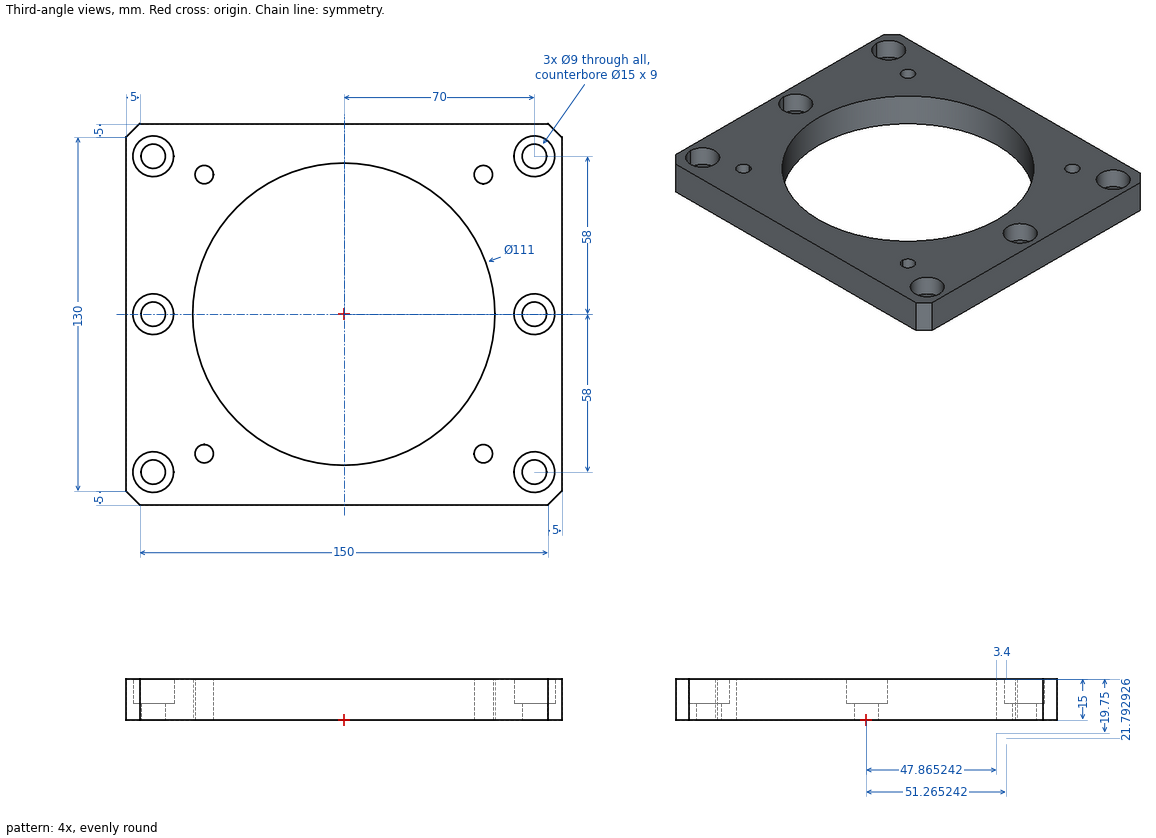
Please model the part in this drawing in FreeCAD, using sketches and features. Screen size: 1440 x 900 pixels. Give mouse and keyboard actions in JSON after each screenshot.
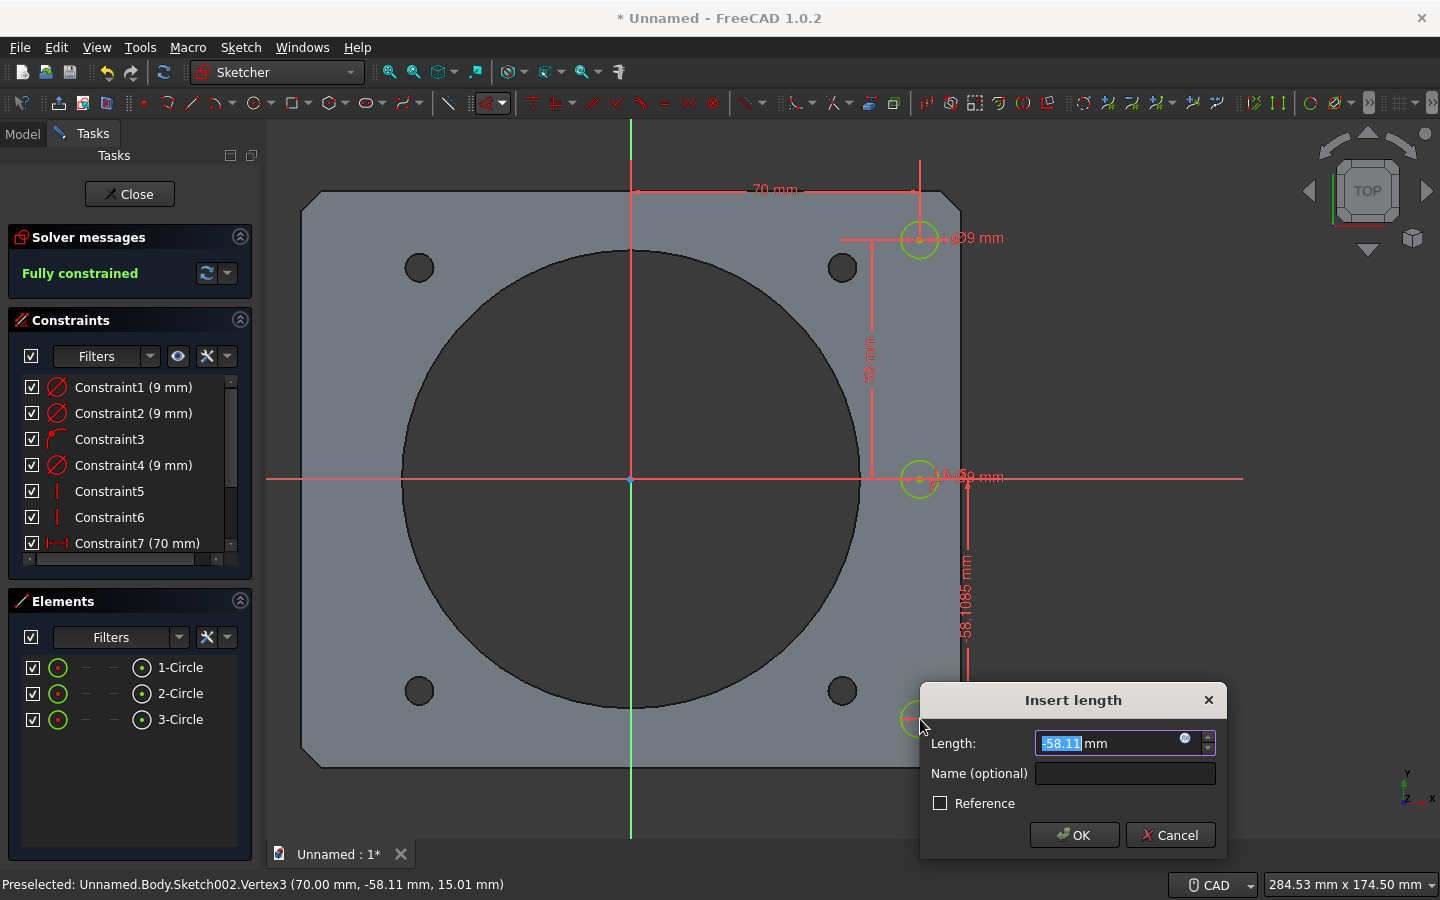
{"action": "type", "text": "-58"}
{"action": "key", "text": "Return"}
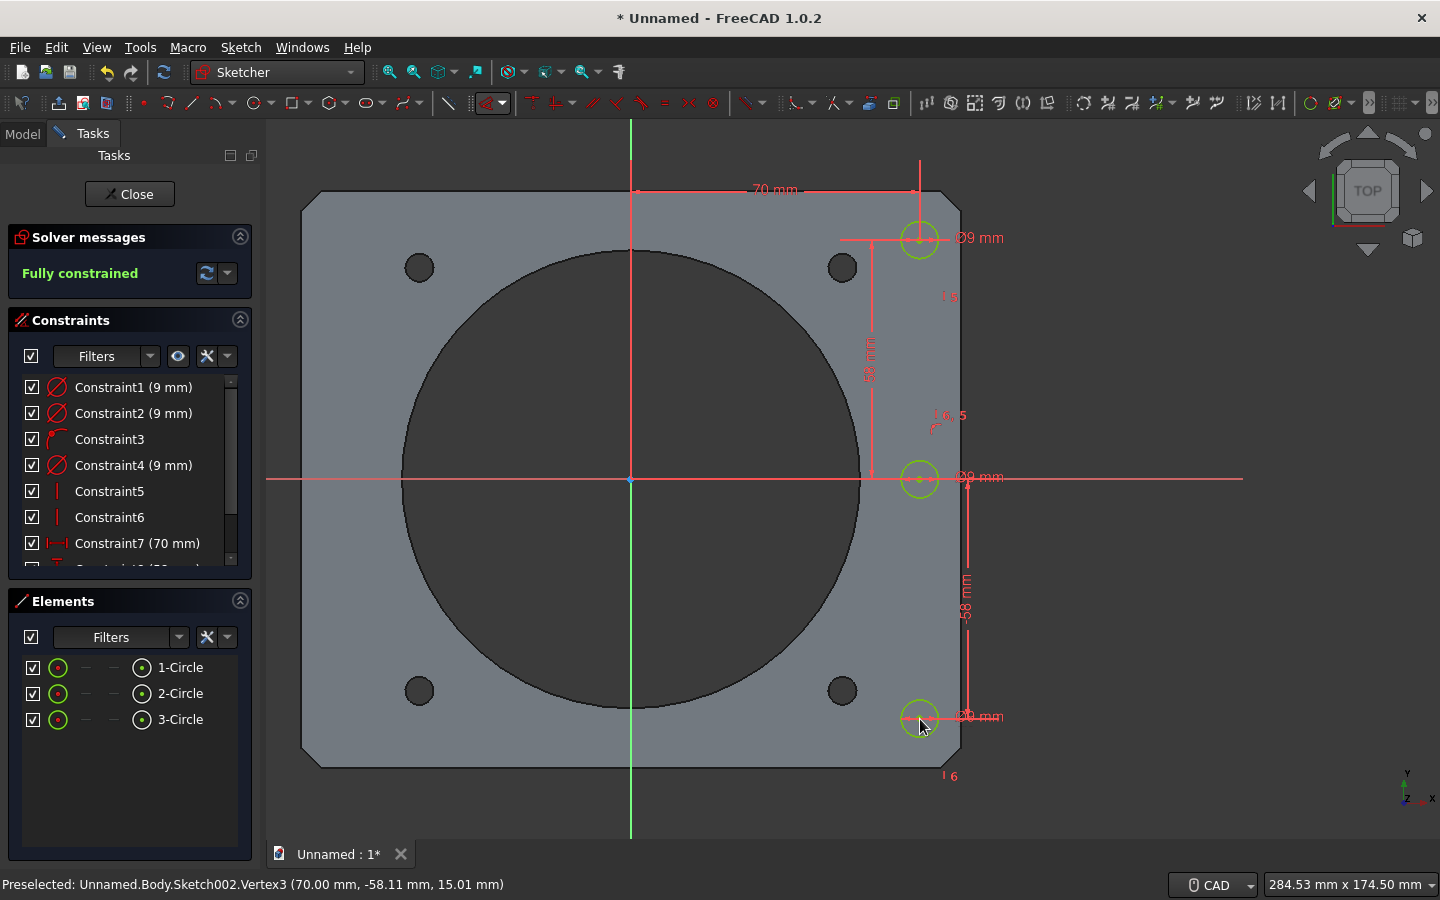
{"action": "left_click", "coordinate": [130, 194]}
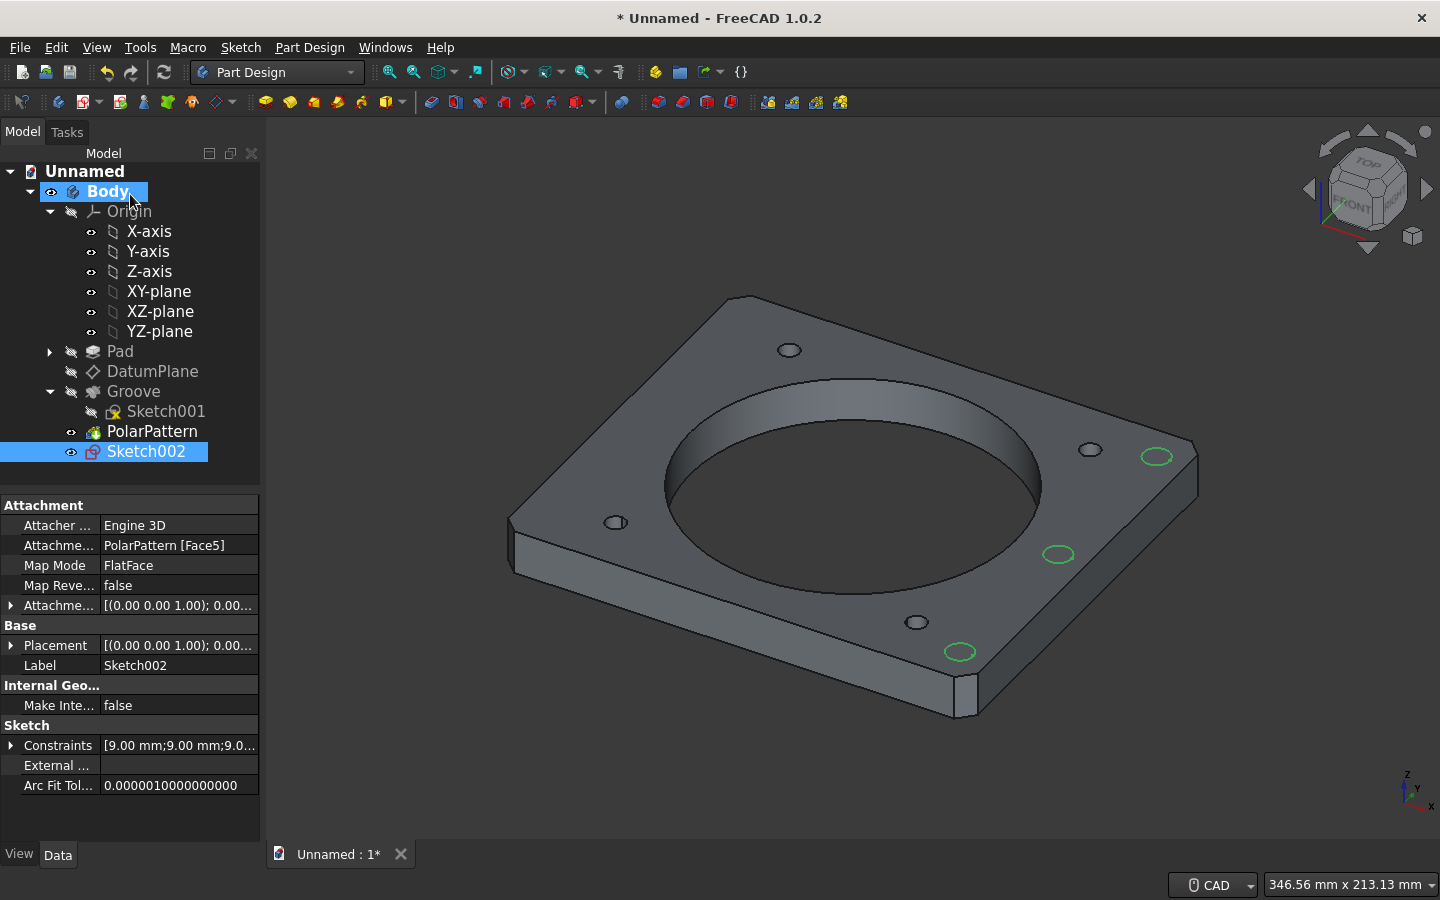
{"action": "left_click", "coordinate": [456, 102]}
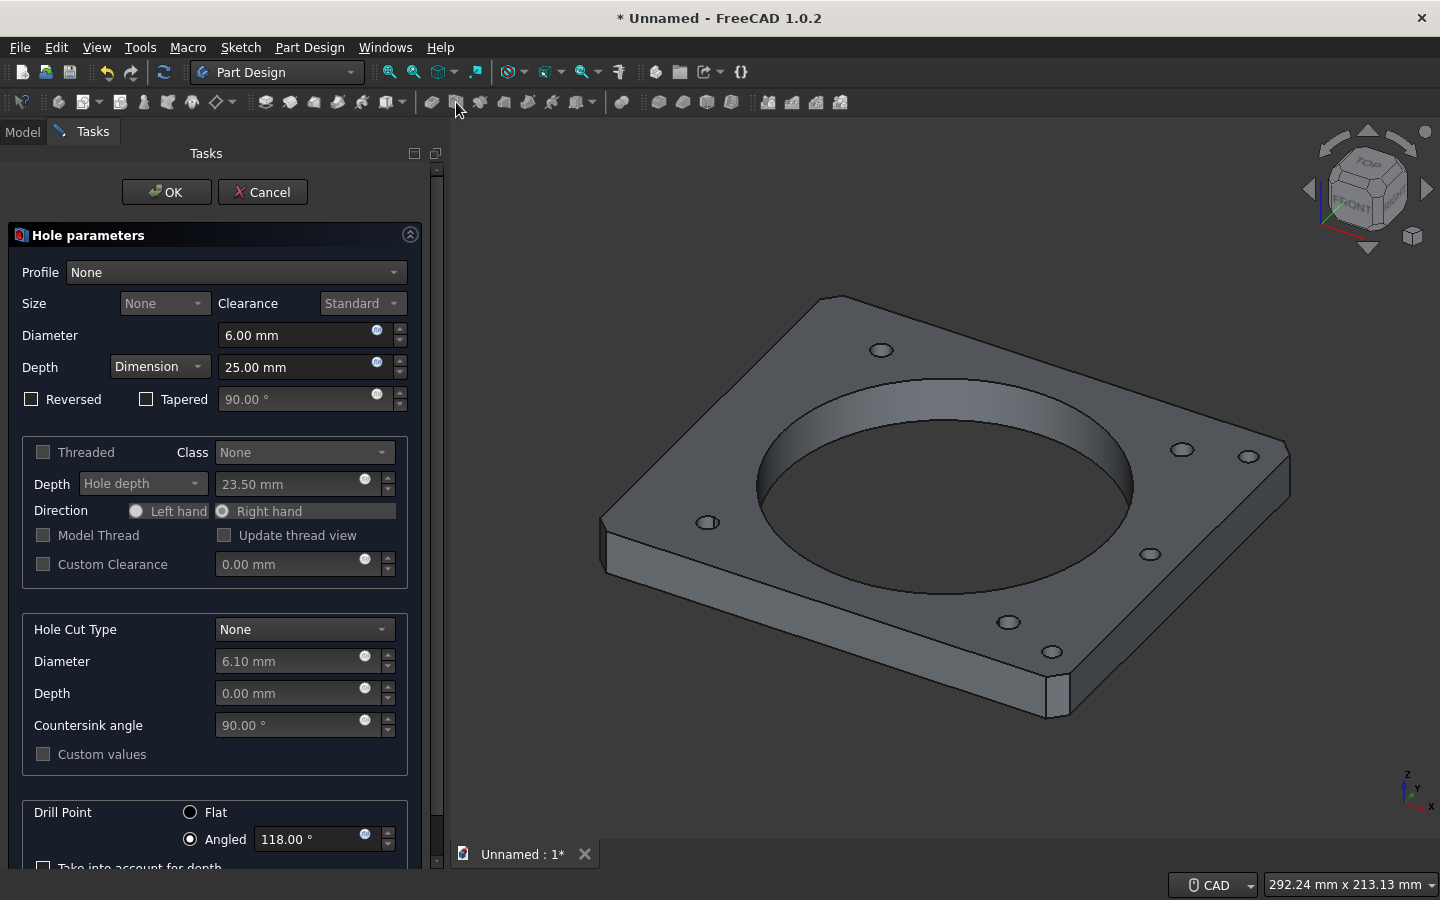
{"action": "triple_click", "coordinate": [305, 335]}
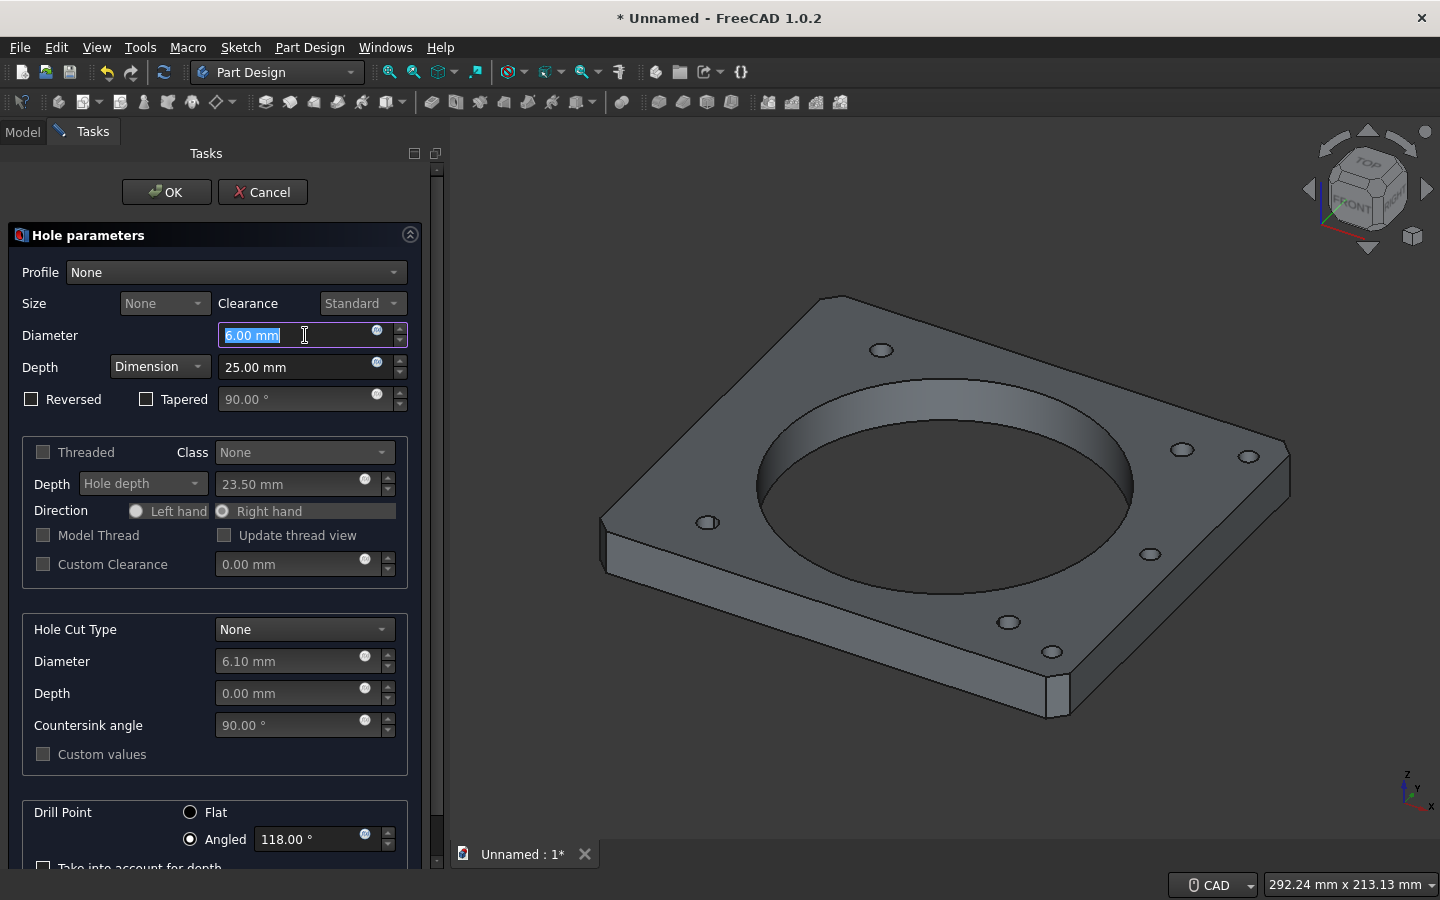
{"action": "type", "text": "9"}
{"action": "key", "text": "Tab"}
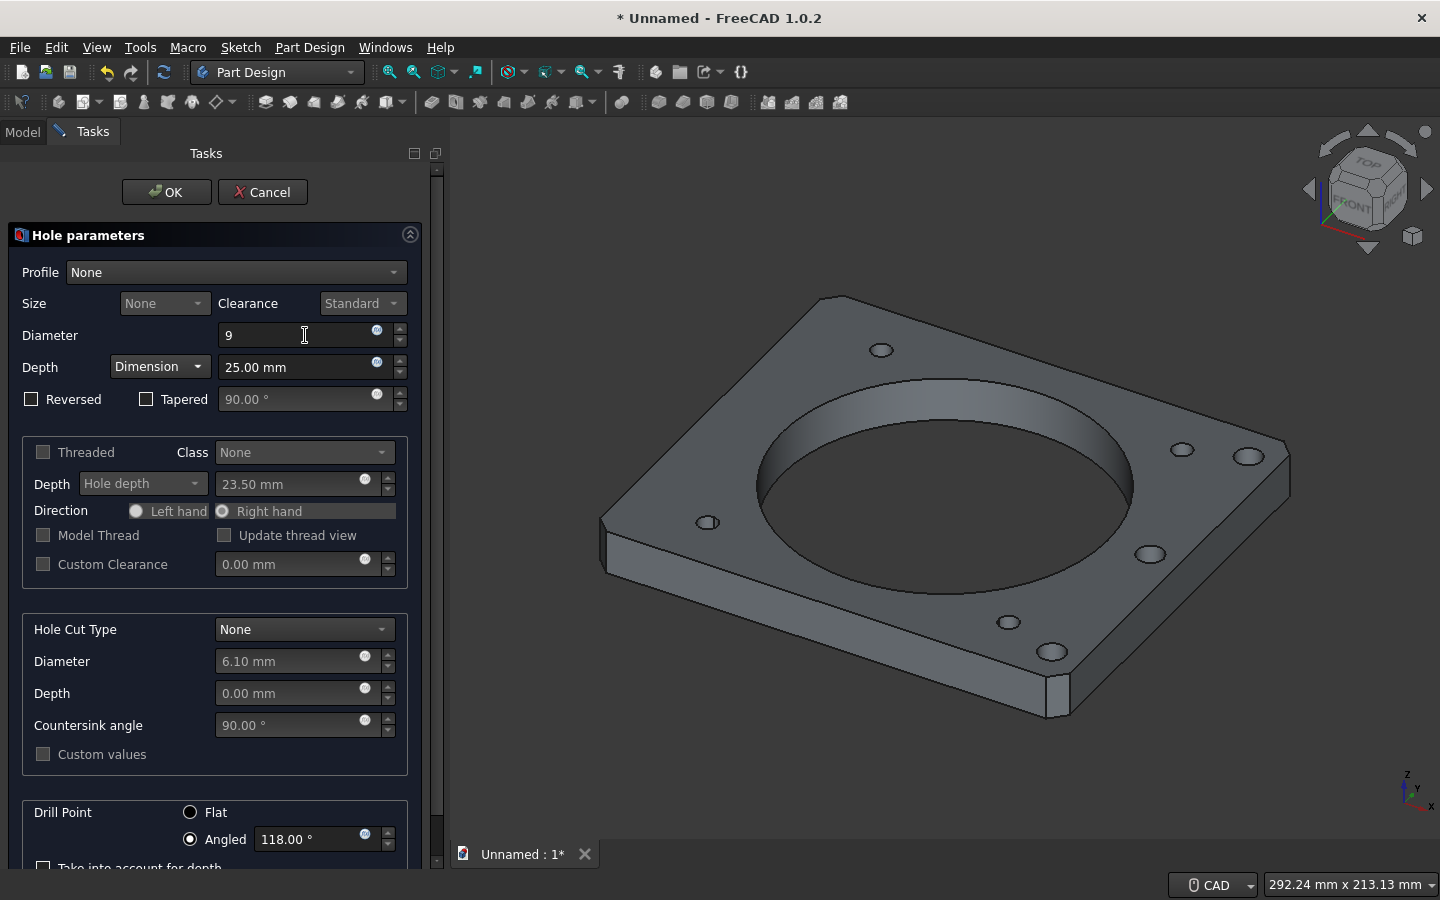
{"action": "left_click", "coordinate": [161, 366]}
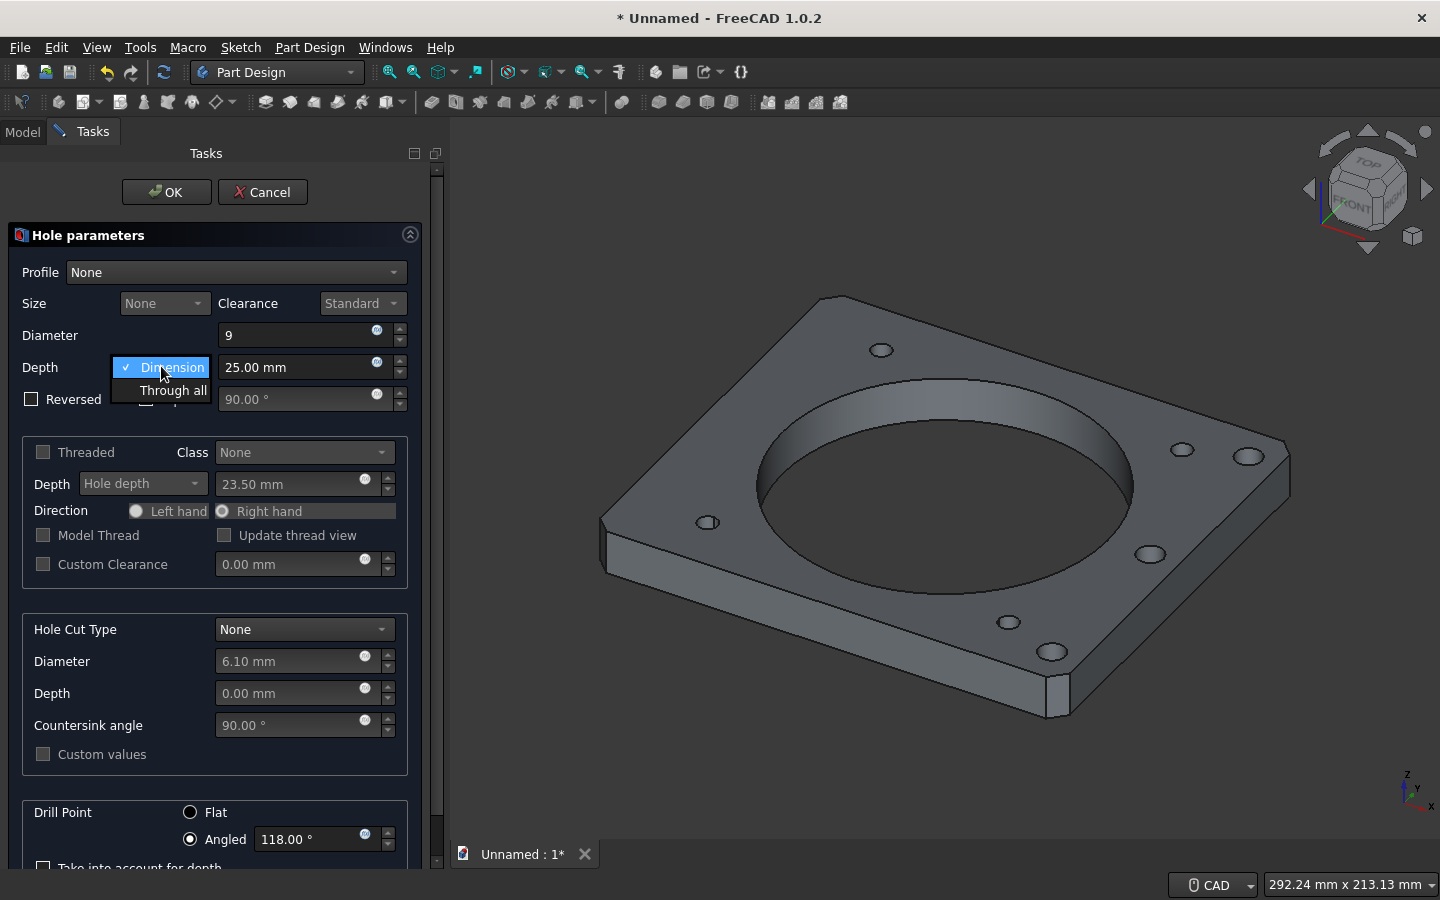
{"action": "left_click", "coordinate": [160, 390]}